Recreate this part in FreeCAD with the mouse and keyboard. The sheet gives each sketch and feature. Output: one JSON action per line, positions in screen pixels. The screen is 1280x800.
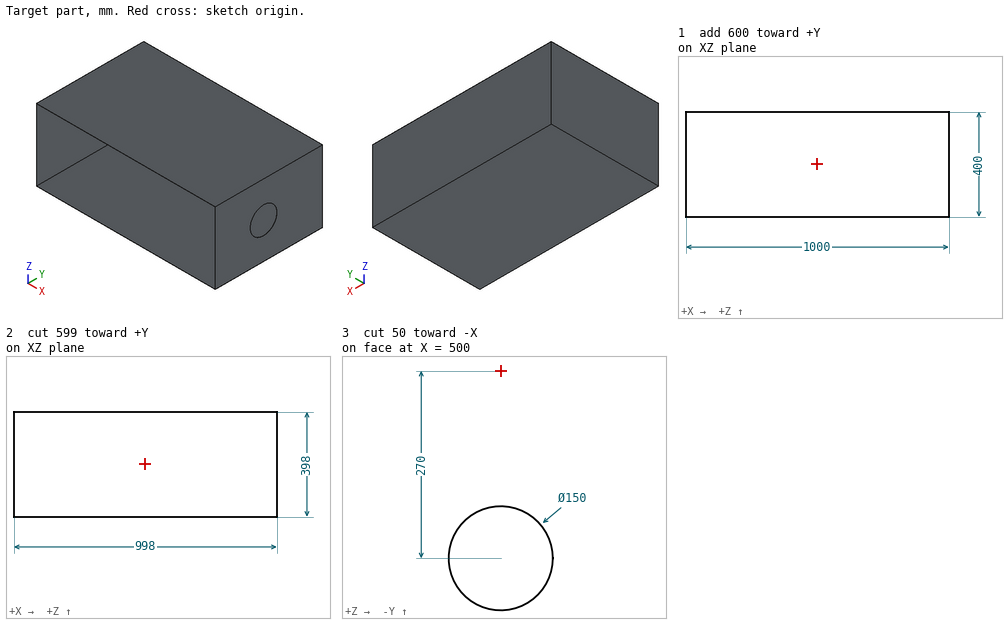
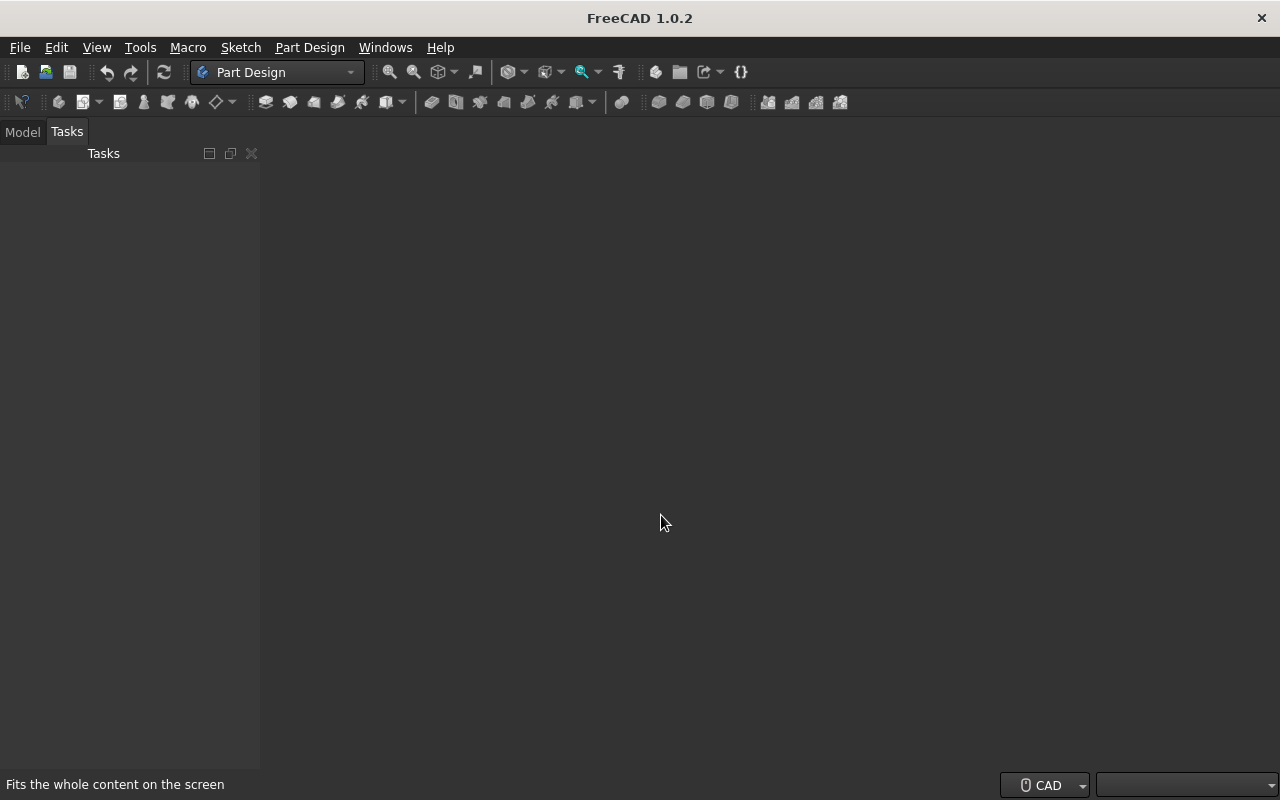
{"action": "key", "text": "ctrl+n"}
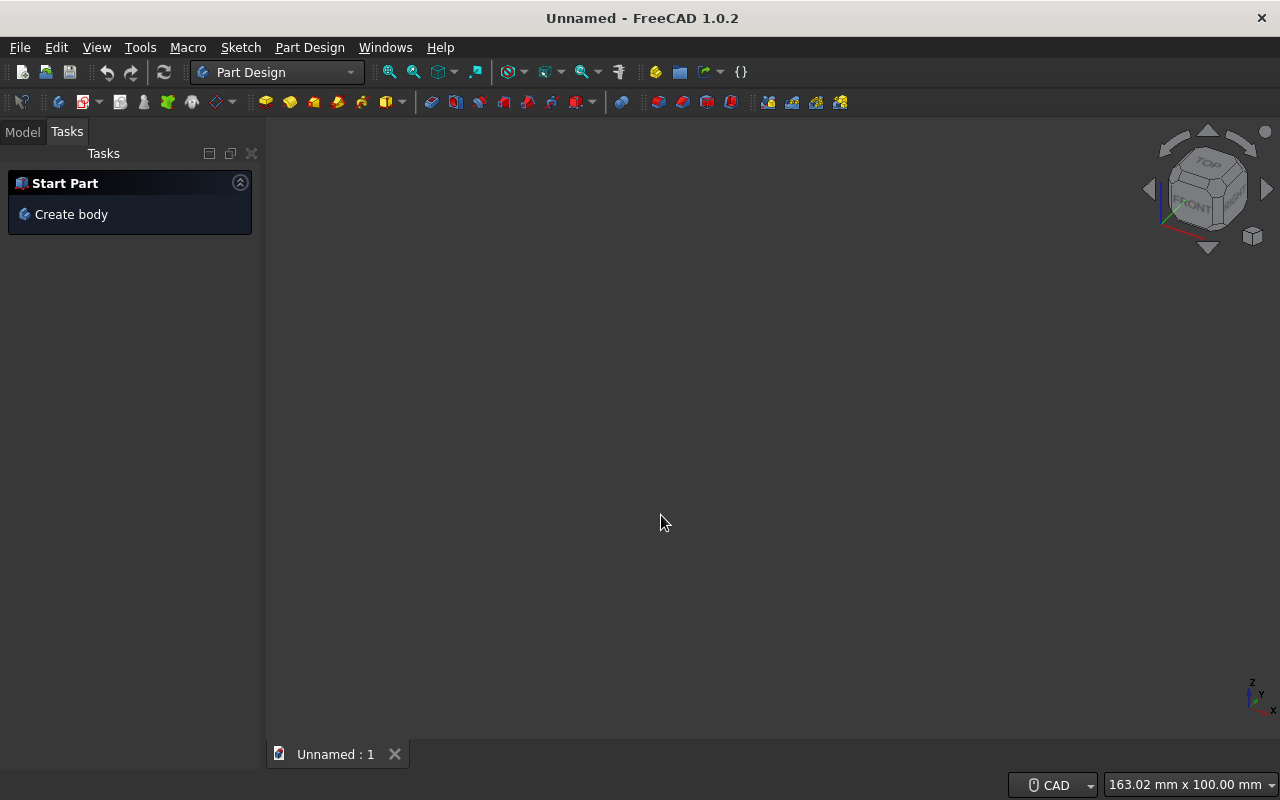
{"action": "left_click", "coordinate": [84, 102]}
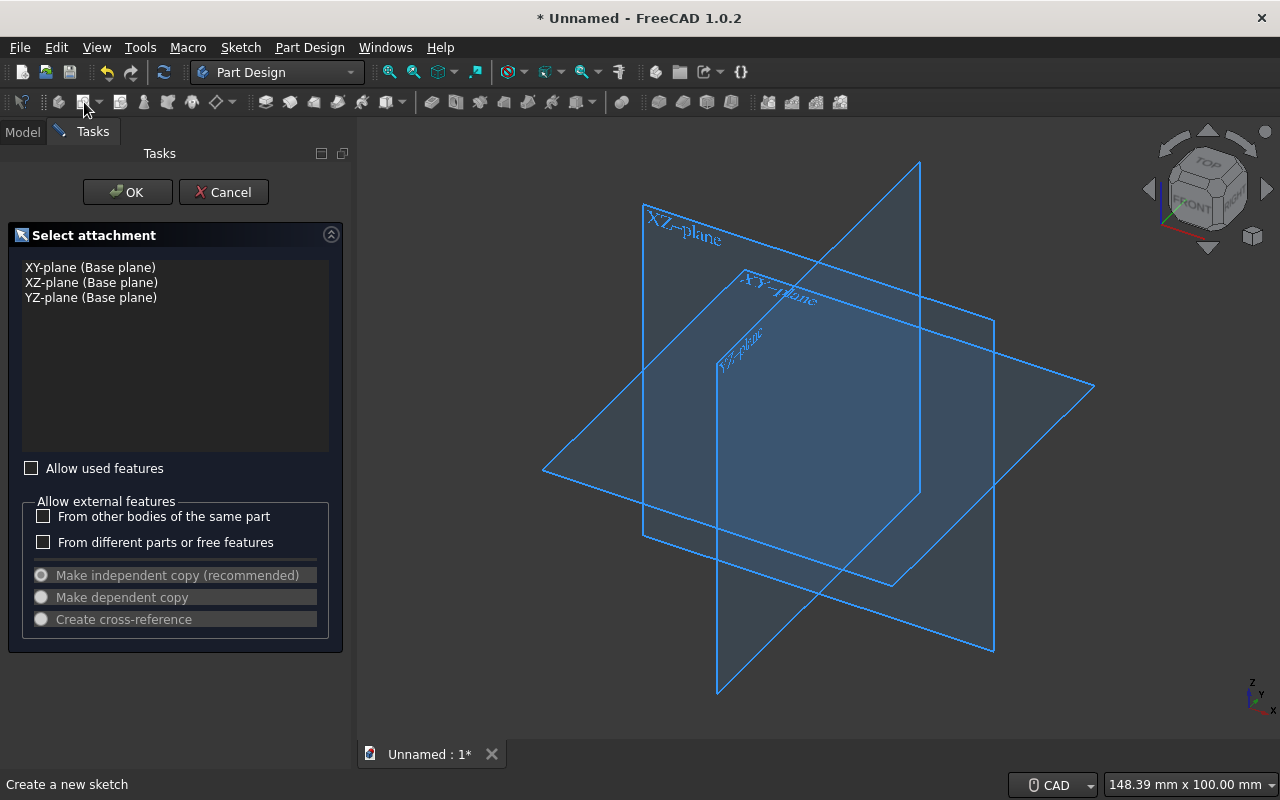
{"action": "left_click", "coordinate": [82, 282]}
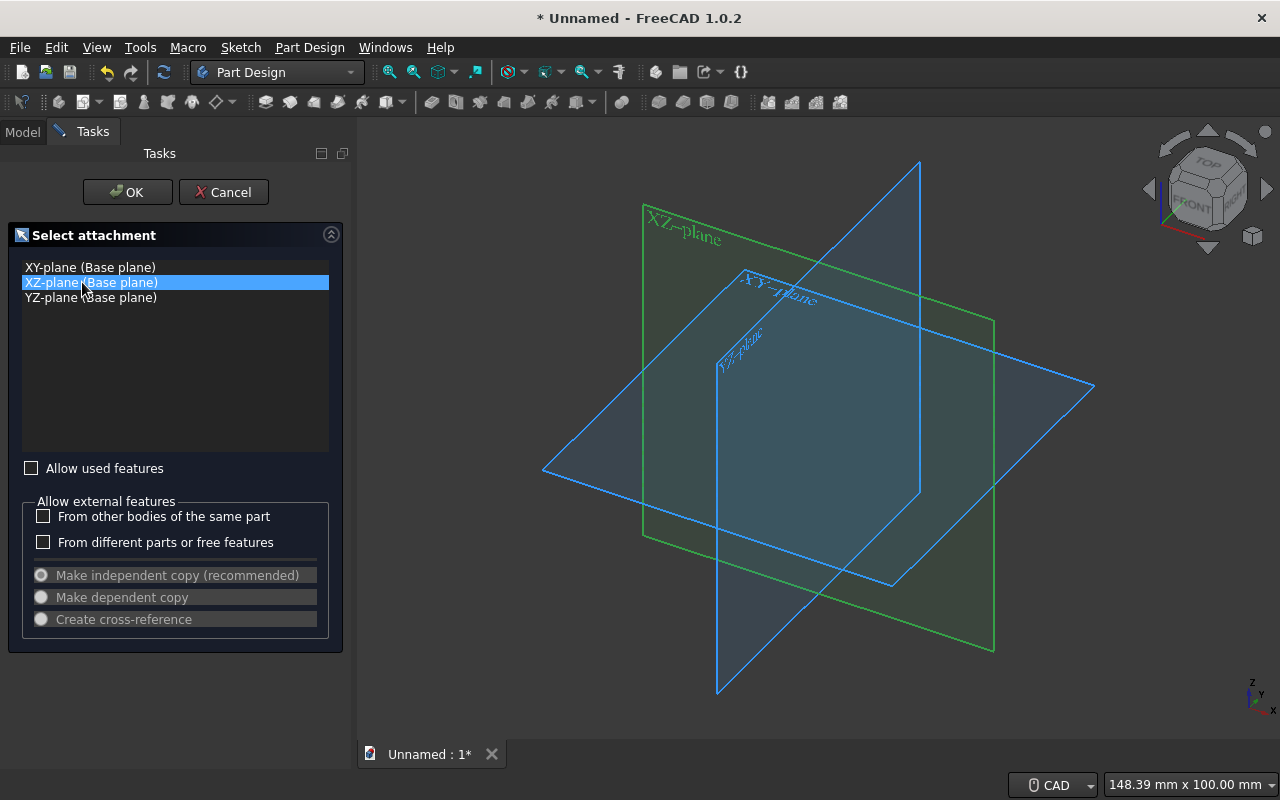
{"action": "left_click", "coordinate": [128, 192]}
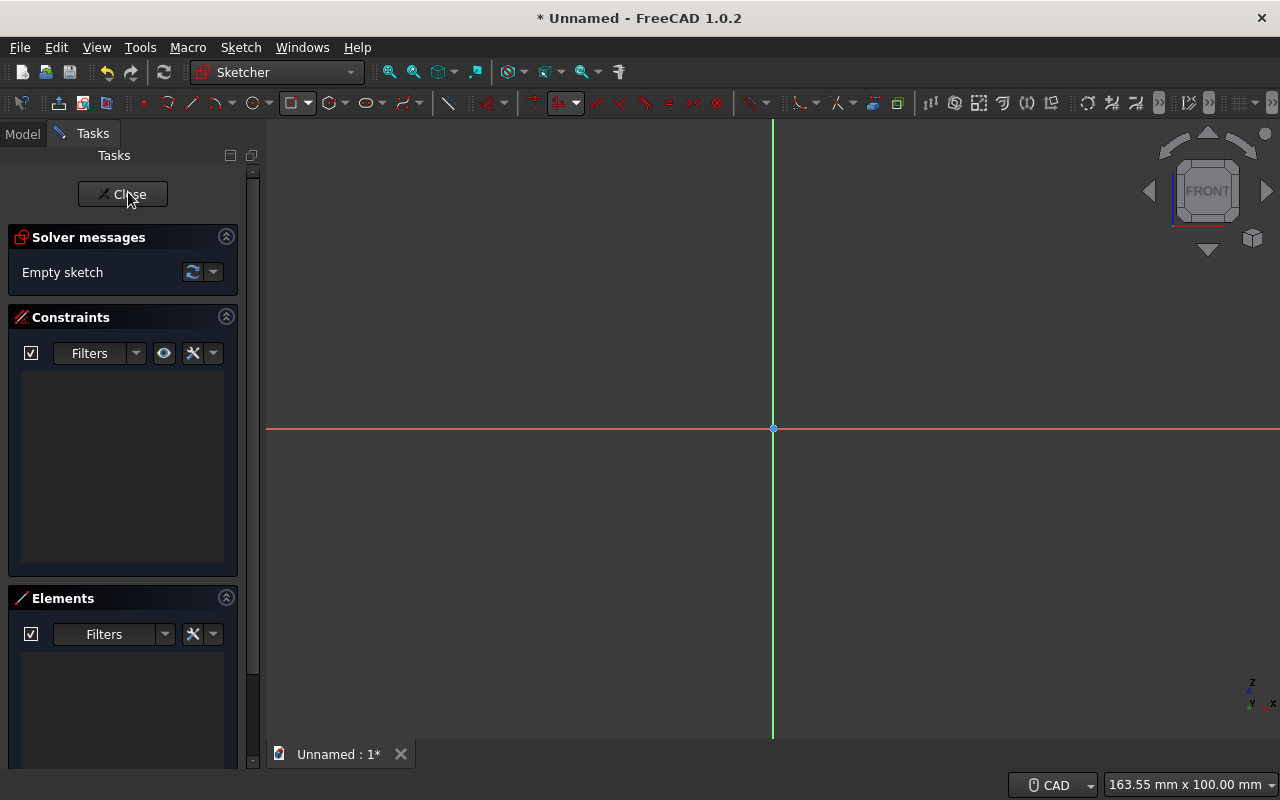
{"action": "scroll", "coordinate": [698, 429], "scroll_direction": "down", "scroll_amount": 12}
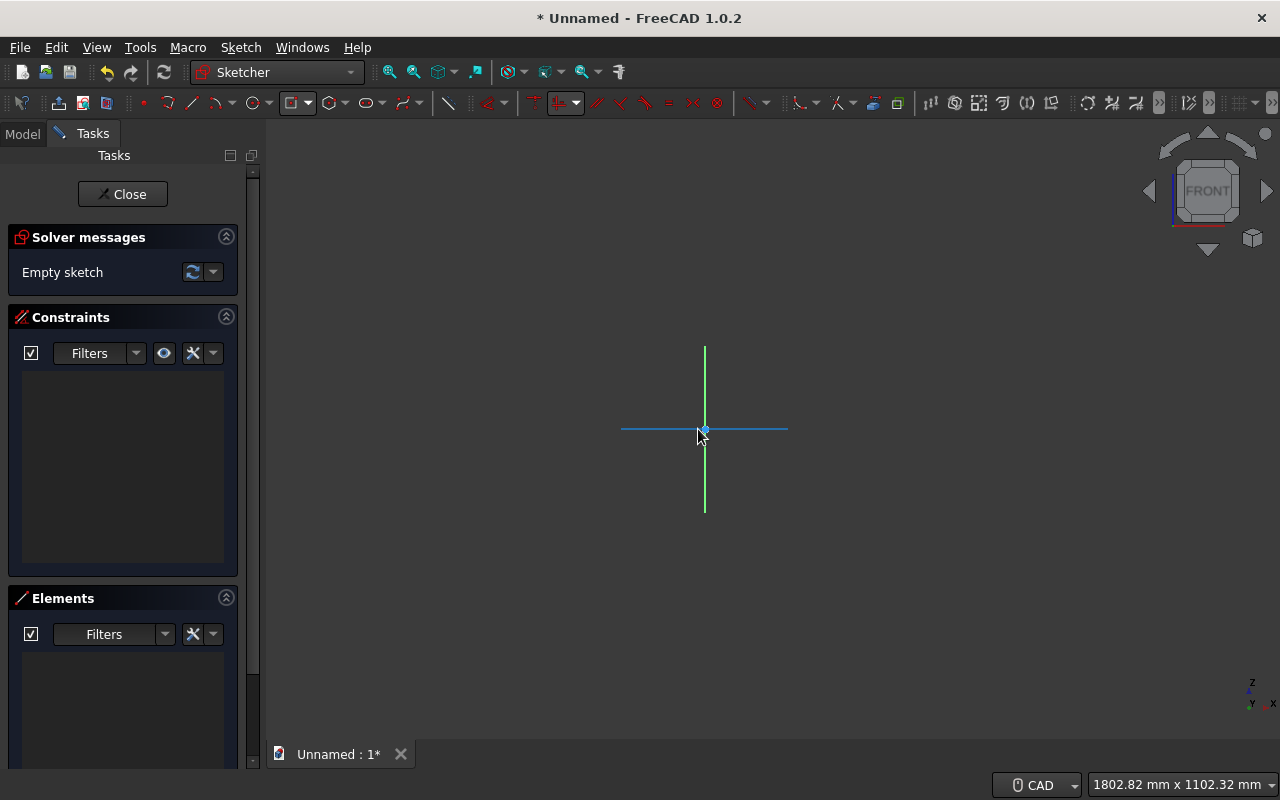
{"action": "key", "text": "g v"}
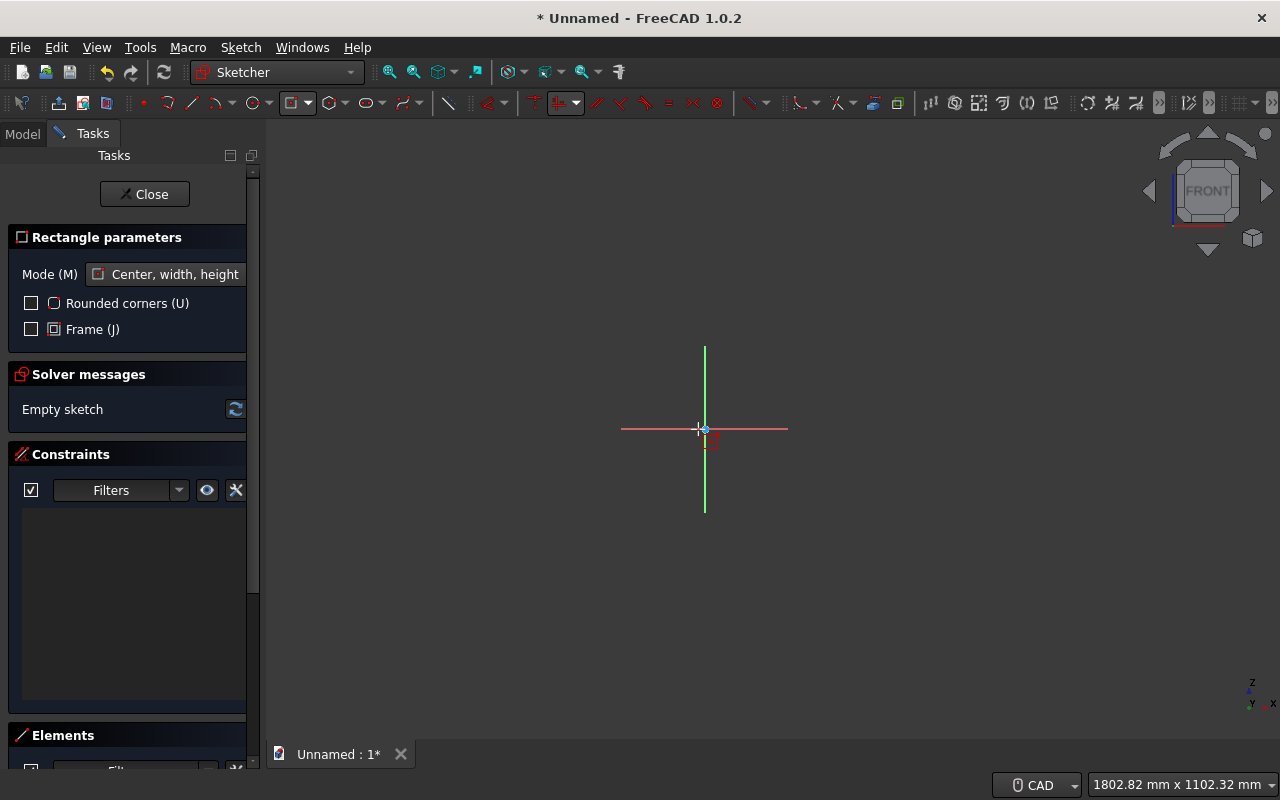
{"action": "left_click", "coordinate": [705, 429]}
{"action": "left_click", "coordinate": [986, 317]}
{"action": "key", "text": "Escape"}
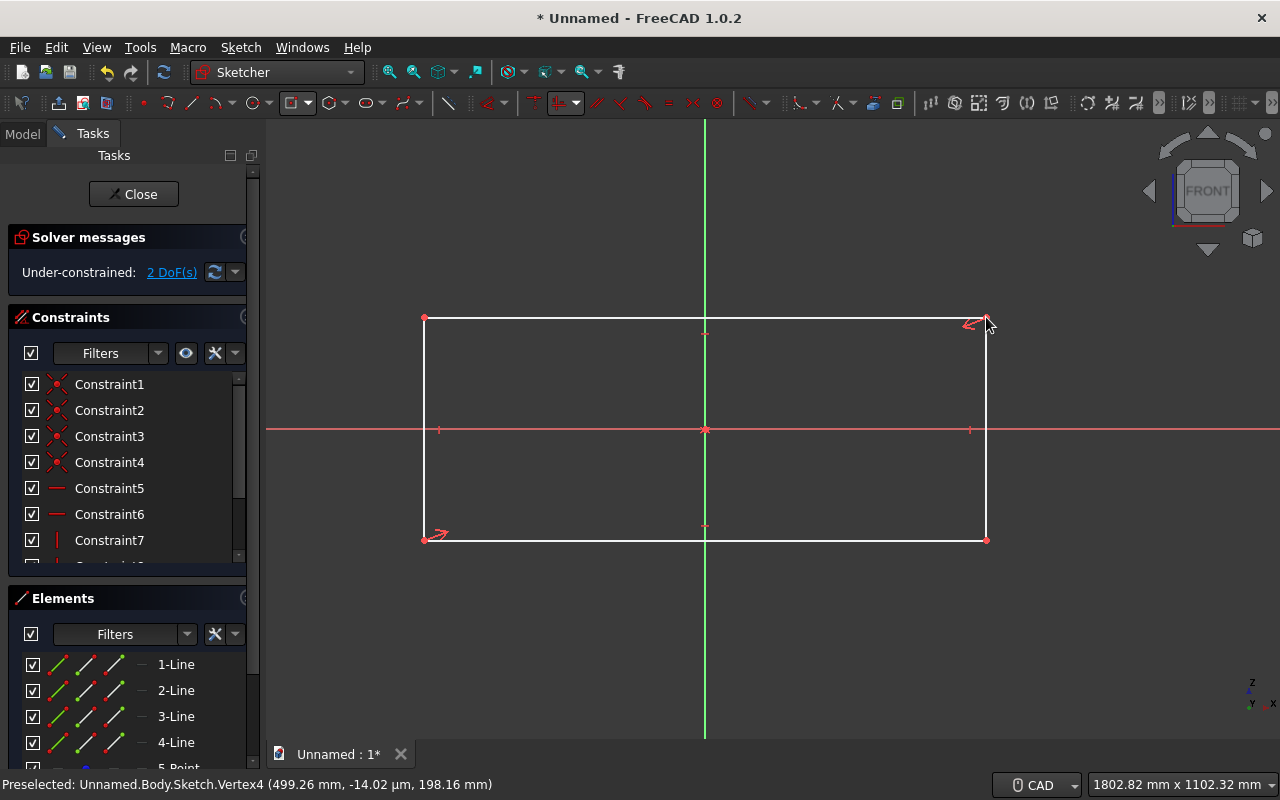
{"action": "key", "text": "d"}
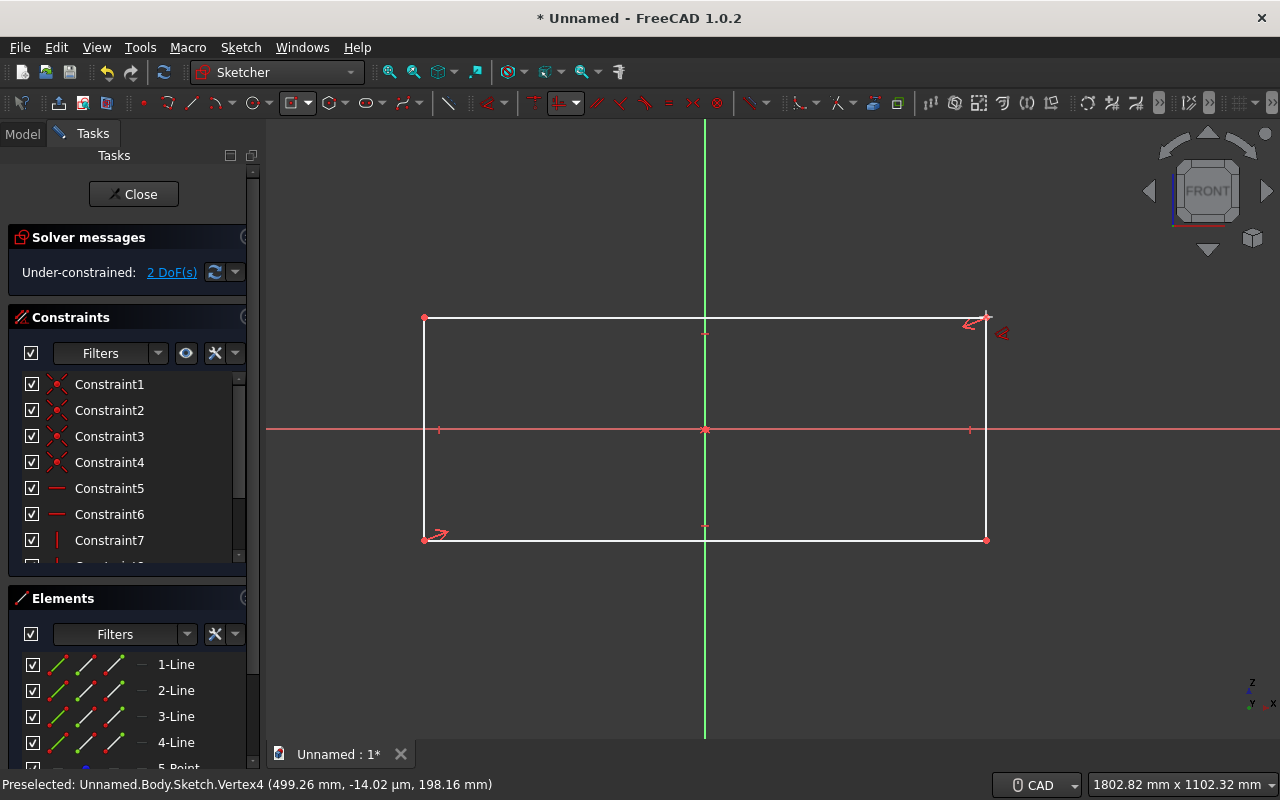
{"action": "left_click", "coordinate": [986, 474]}
{"action": "left_click", "coordinate": [1020, 378]}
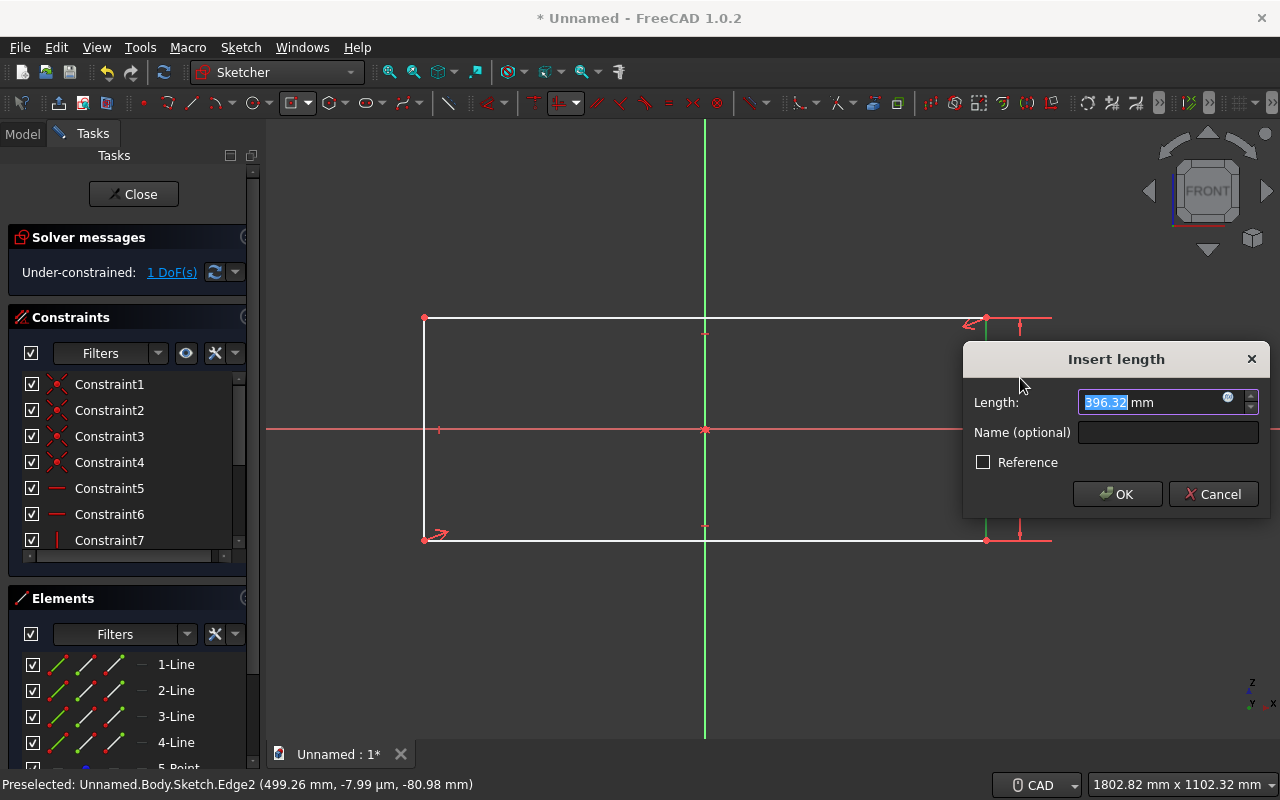
{"action": "type", "text": "400"}
{"action": "key", "text": "Return"}